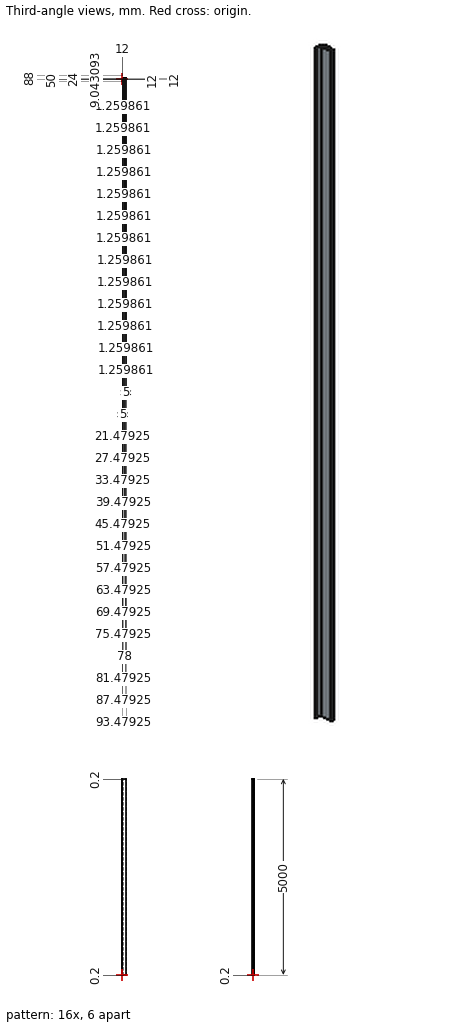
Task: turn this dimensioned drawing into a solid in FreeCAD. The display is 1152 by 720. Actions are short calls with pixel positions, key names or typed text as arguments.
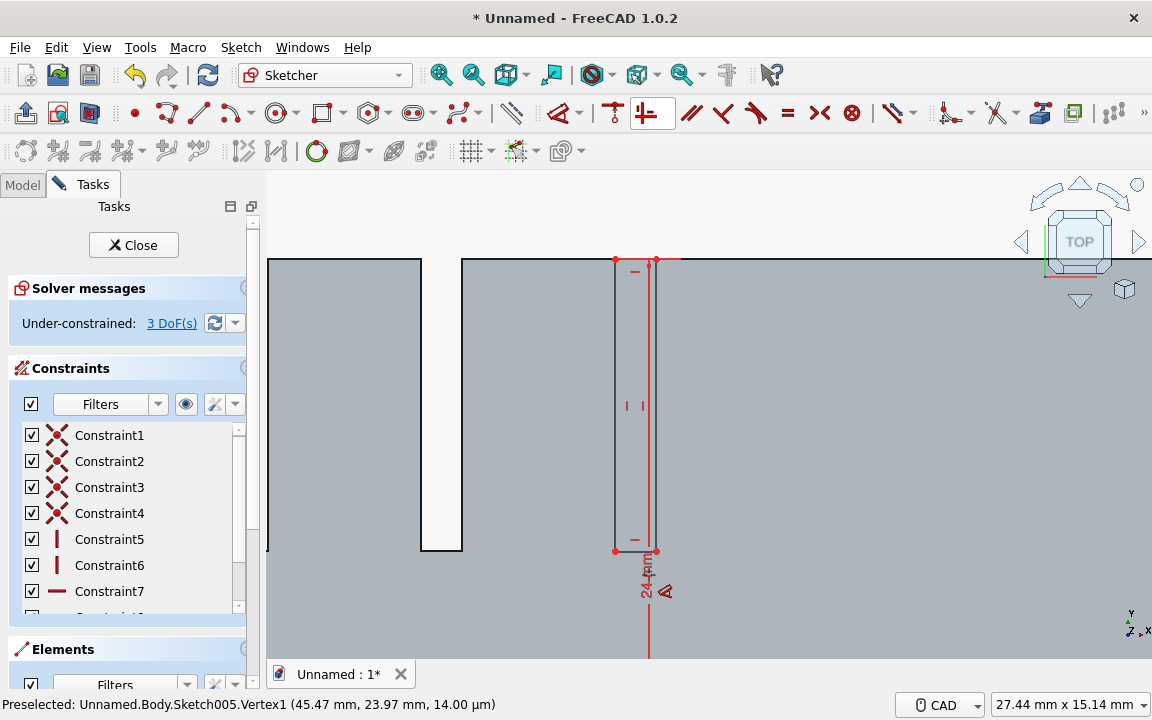
click(615, 347)
click(581, 406)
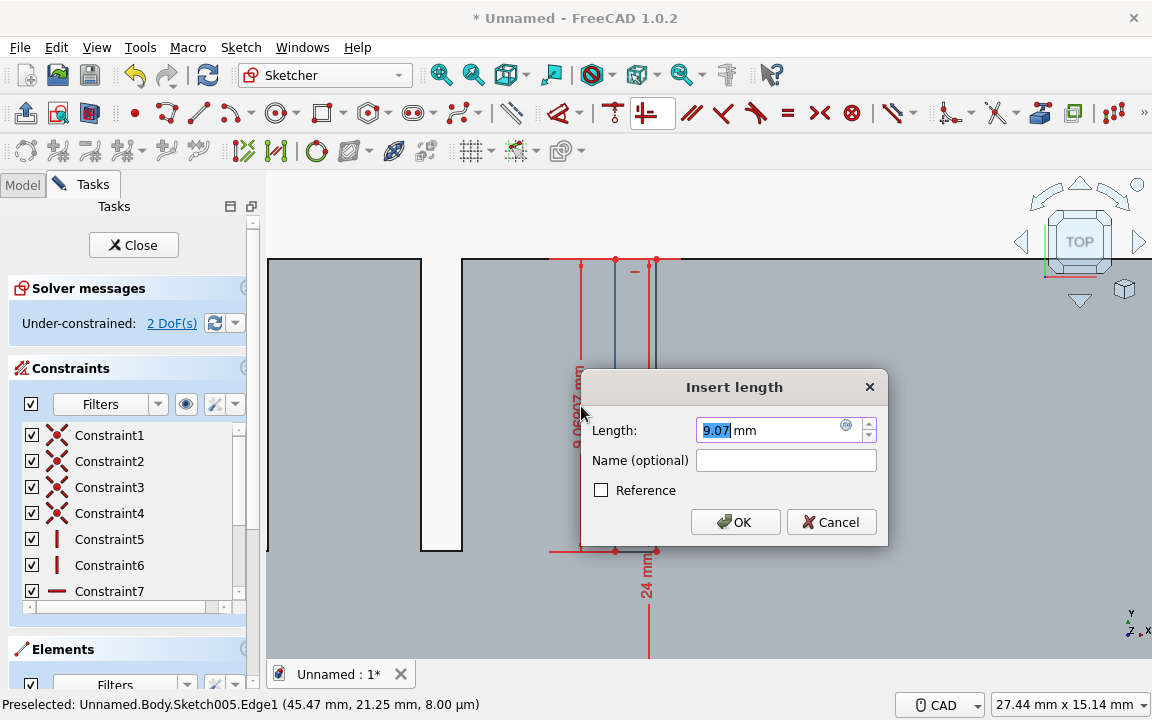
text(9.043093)
key(Return)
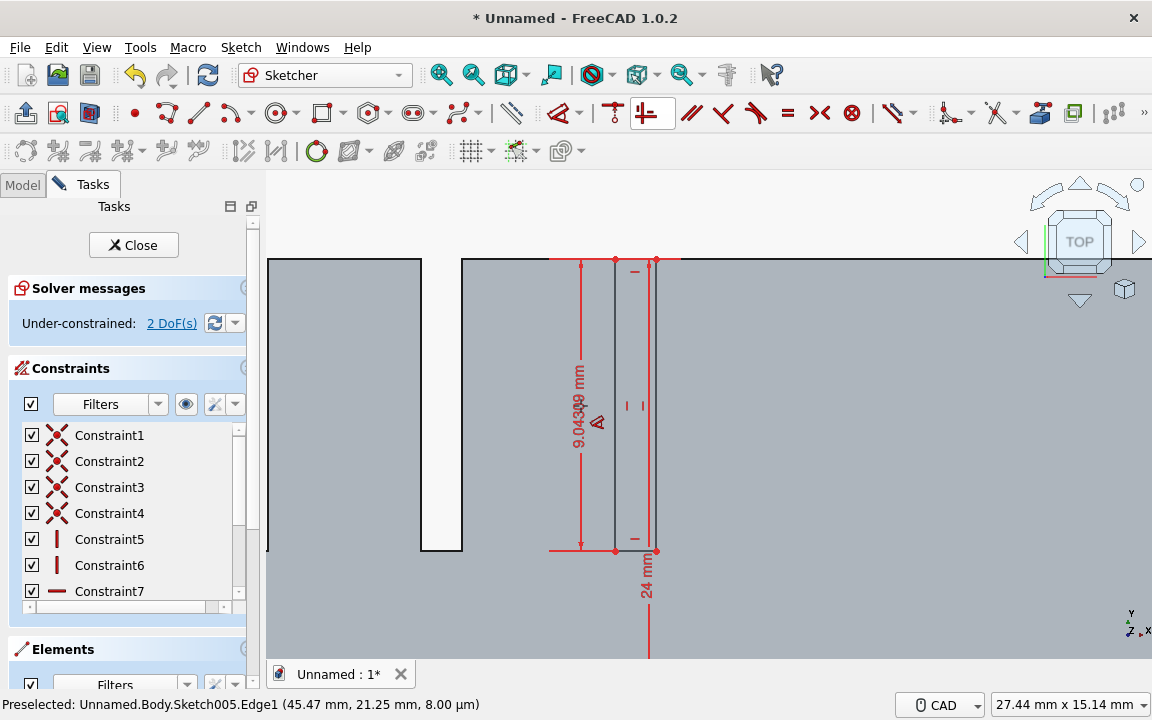
click(627, 551)
click(636, 517)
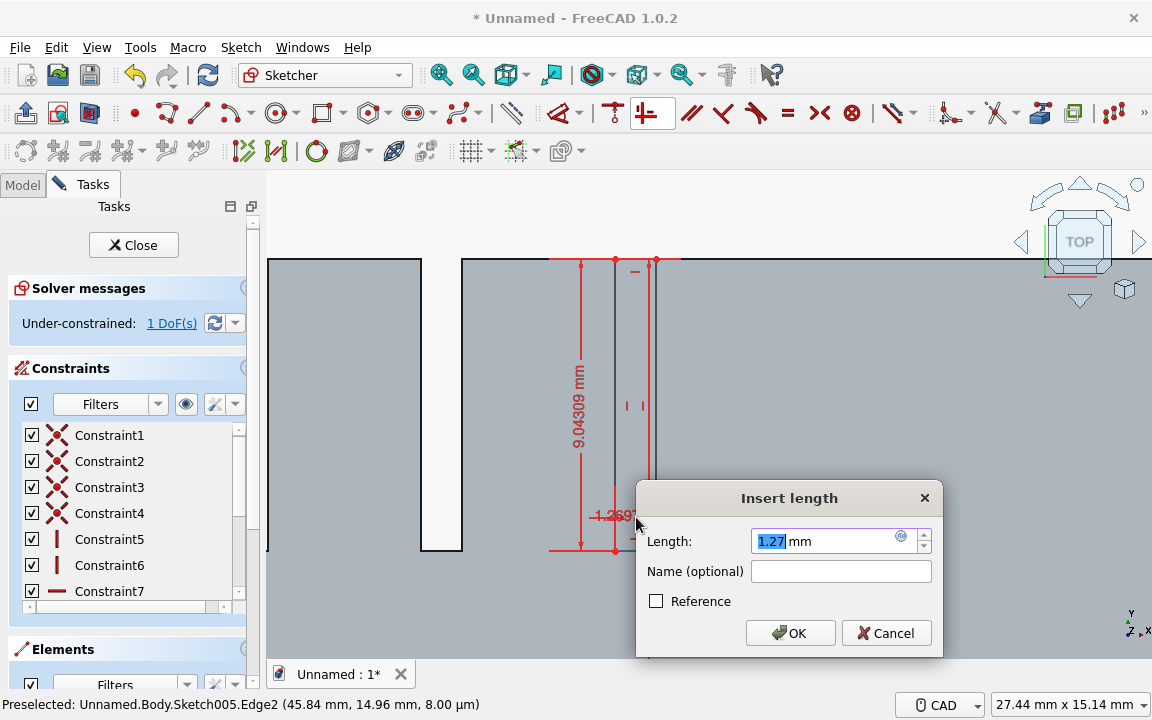
text(1.259861)
key(Return)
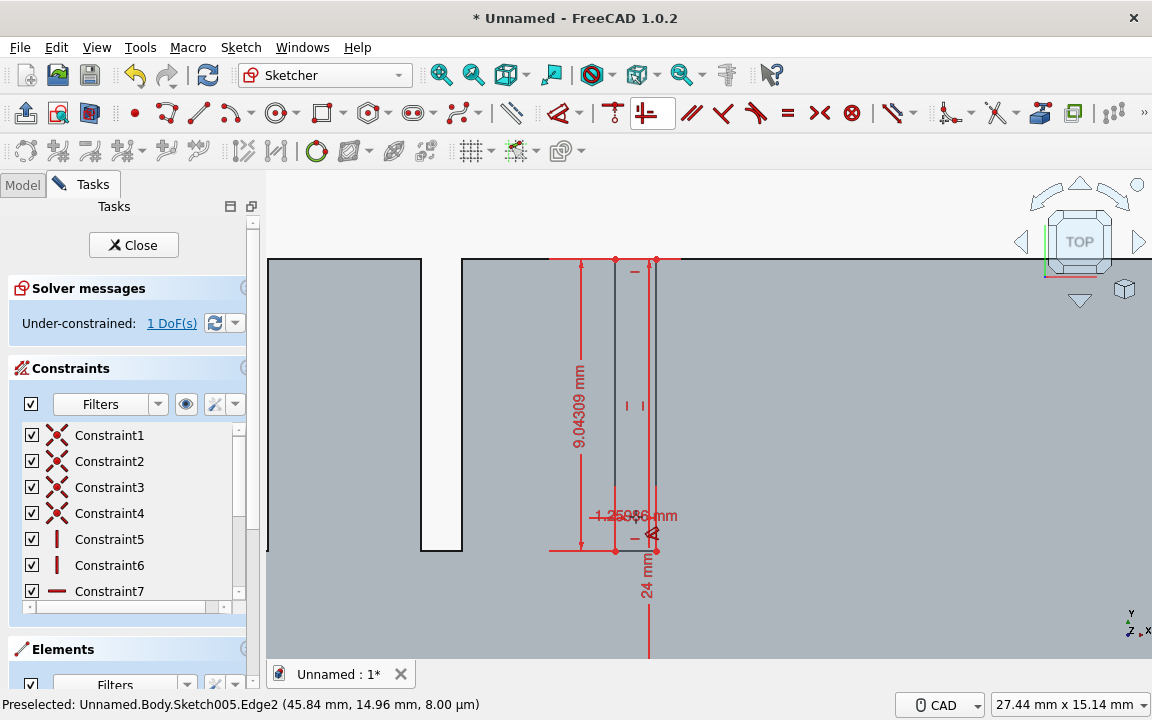
click(615, 259)
click(455, 225)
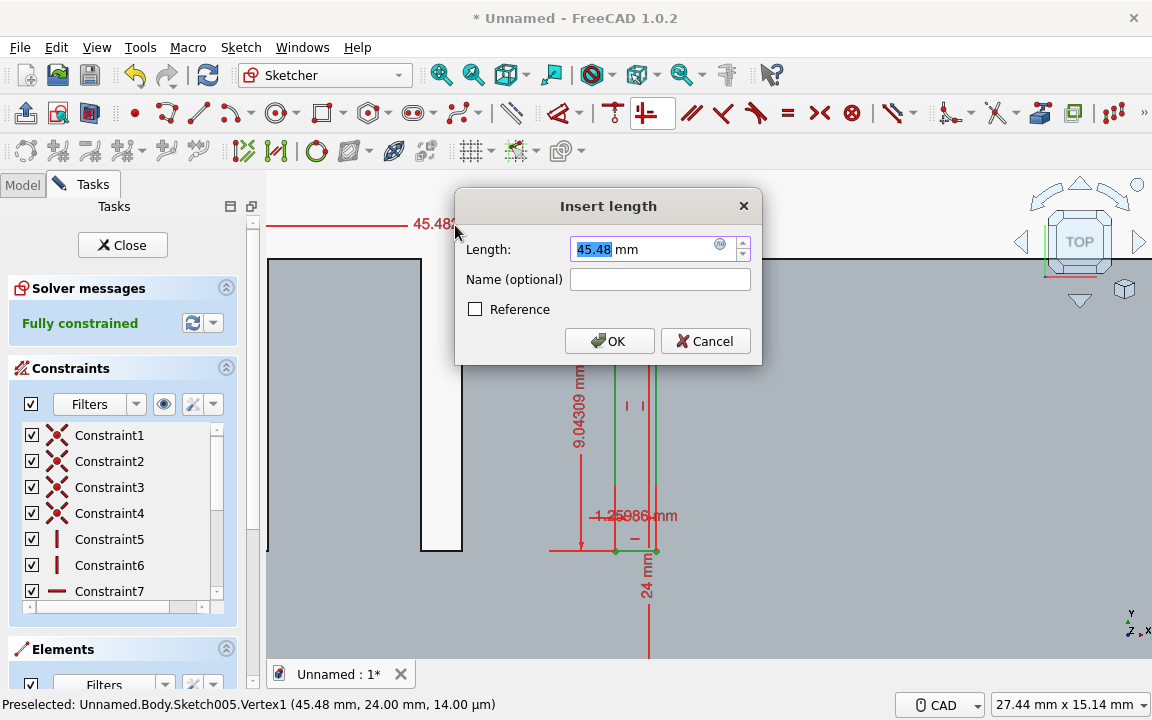
text(45.47925)
key(Return)
key(Escape)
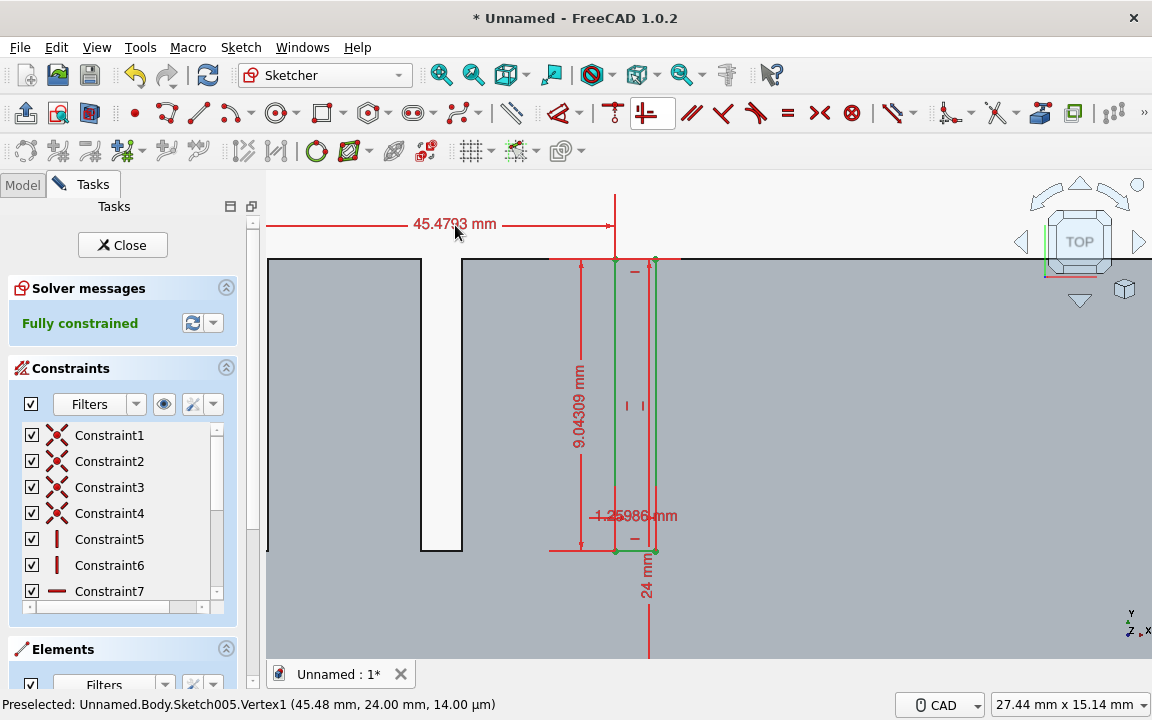
click(123, 245)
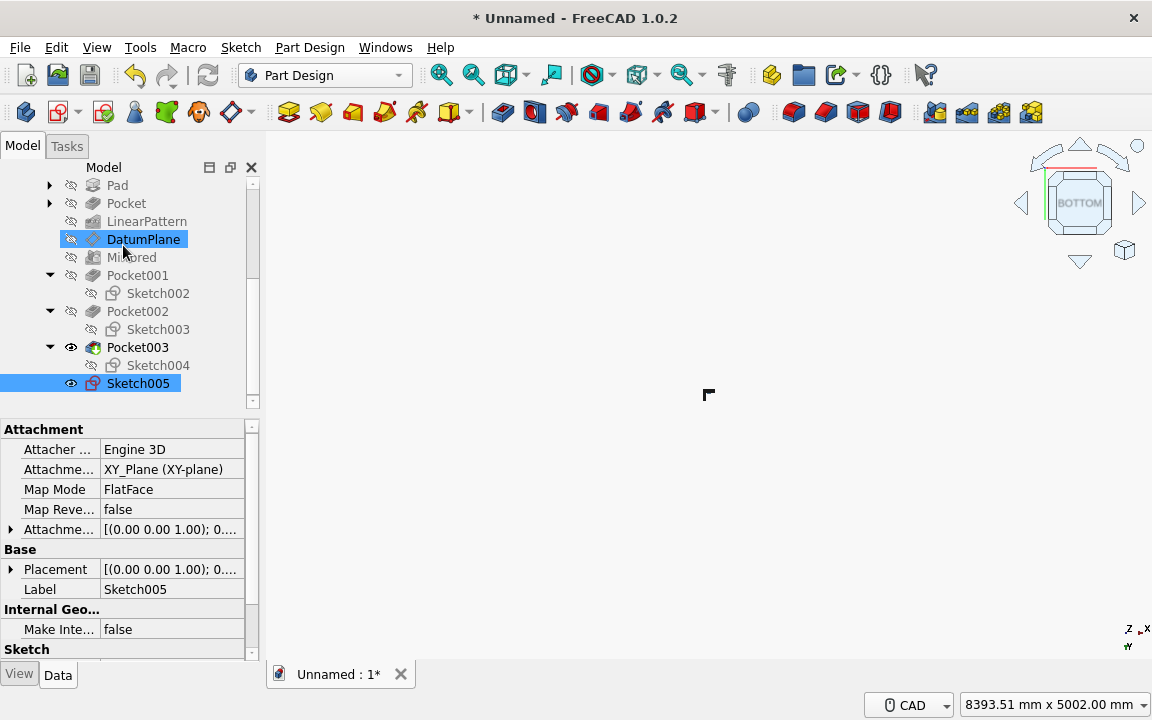
click(504, 112)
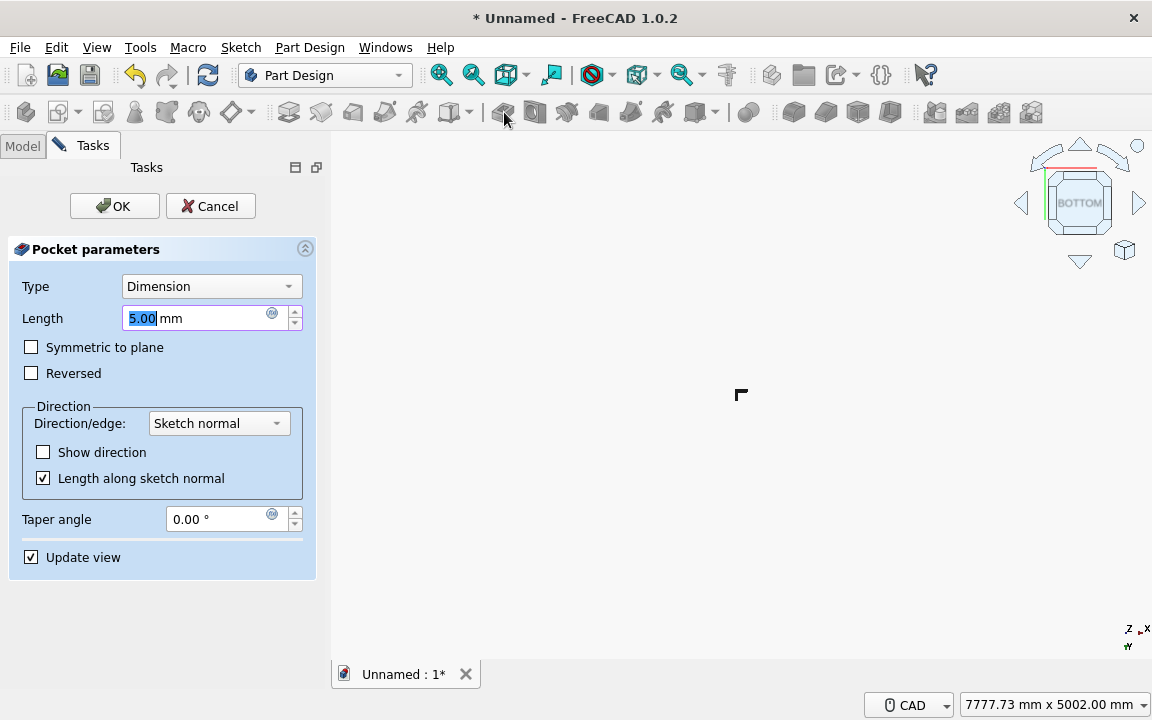
text(0.2)
key(Tab)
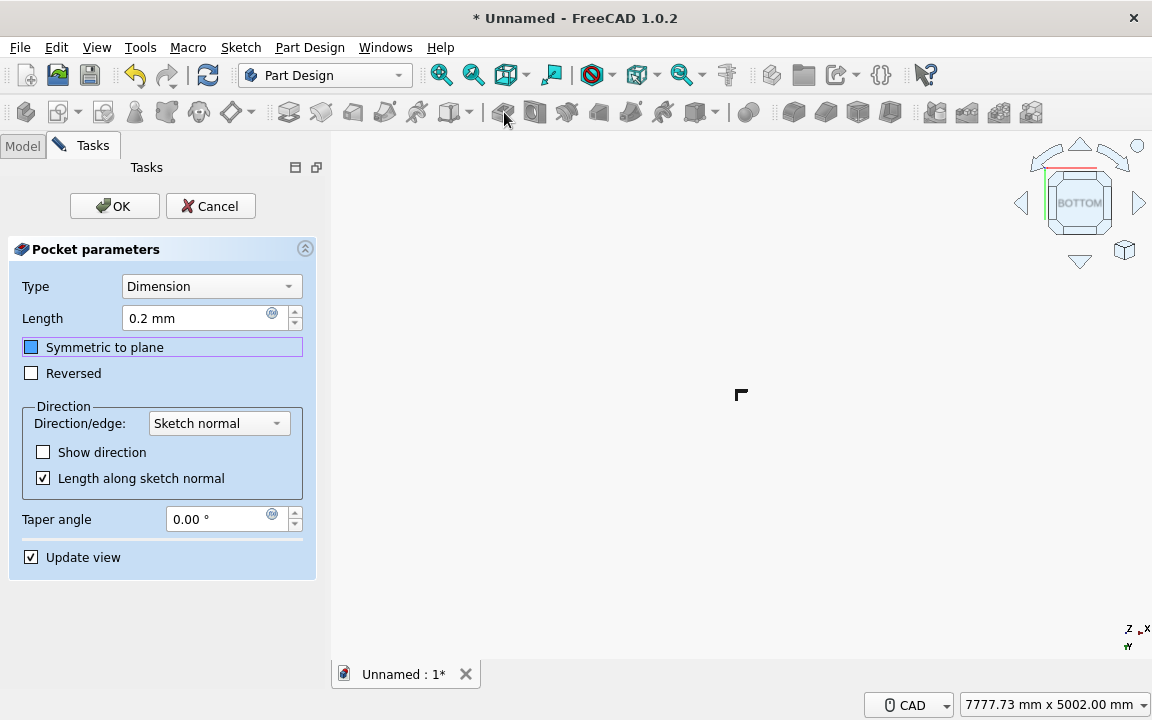
click(30, 373)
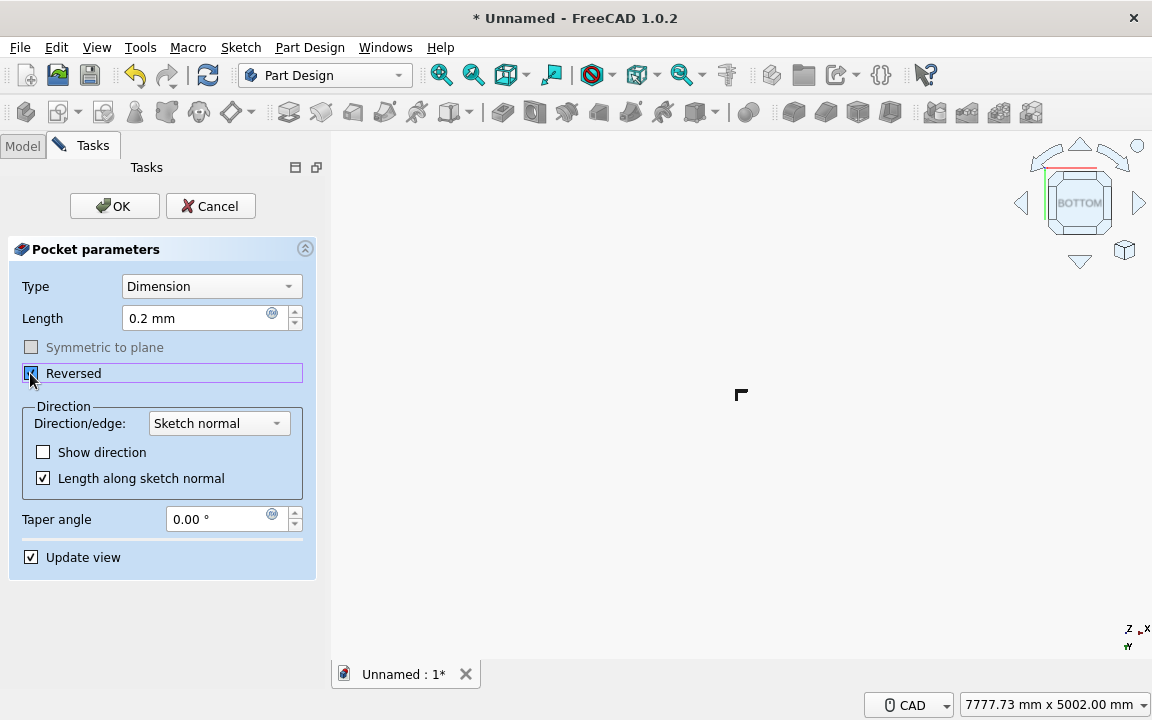
click(115, 206)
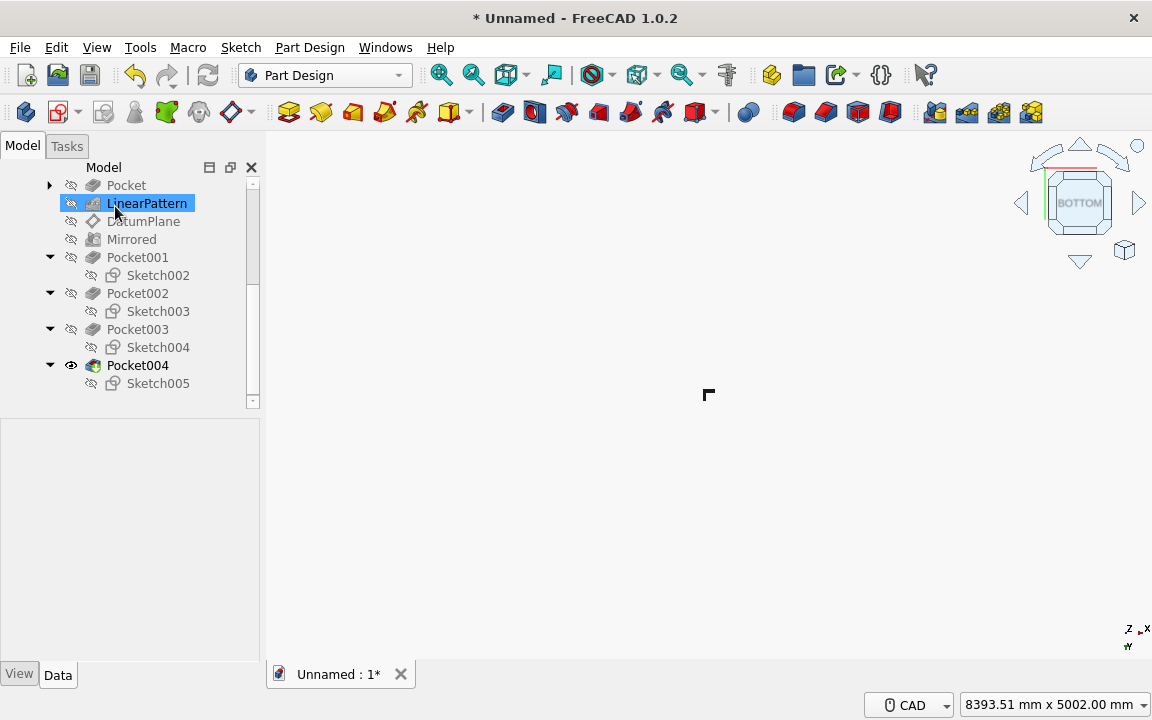
click(442, 76)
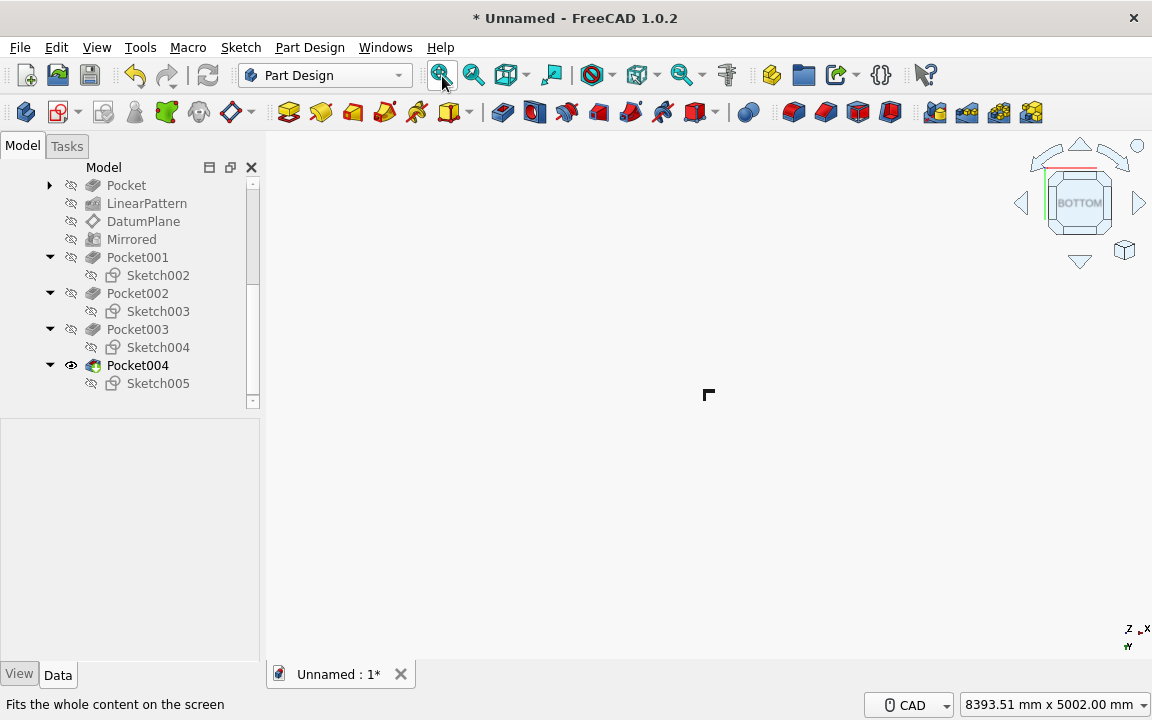
scroll(712, 389, up, 14)